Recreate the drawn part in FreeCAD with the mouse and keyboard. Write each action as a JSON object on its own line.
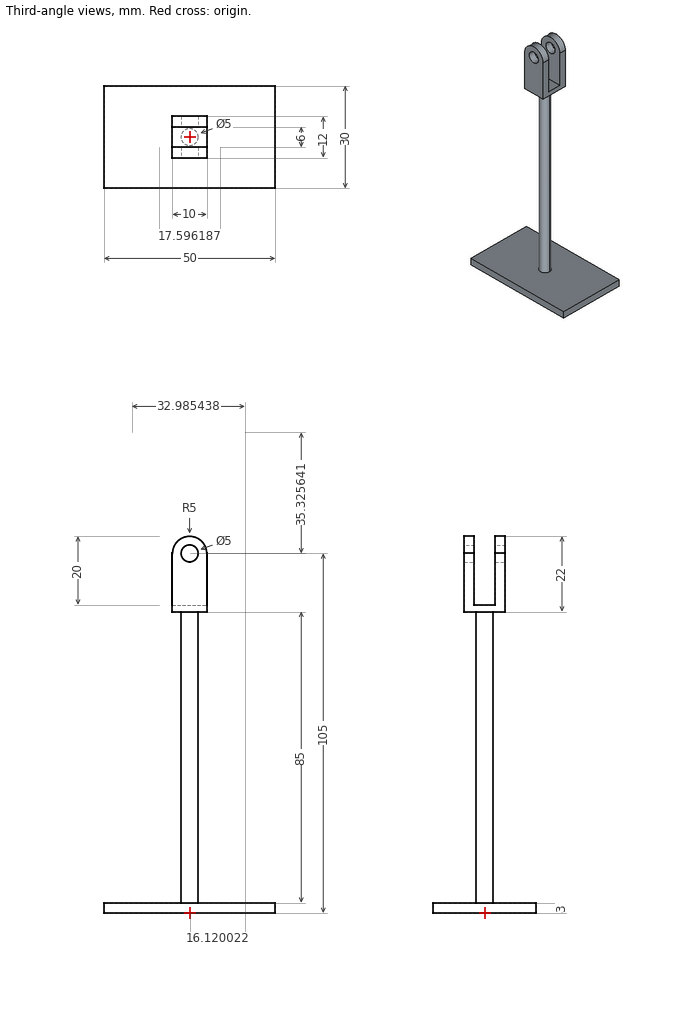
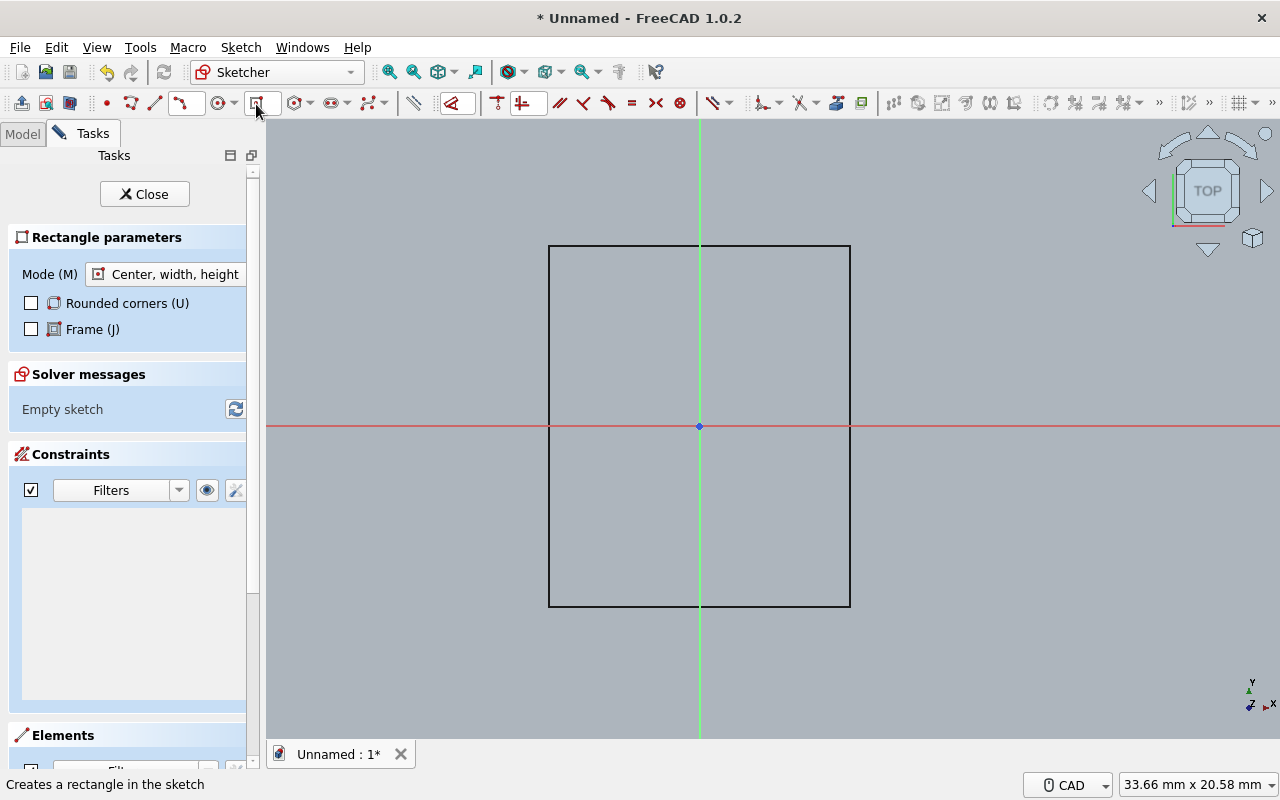
{"action": "left_click", "coordinate": [700, 426]}
{"action": "mouse_move", "coordinate": [965, 336]}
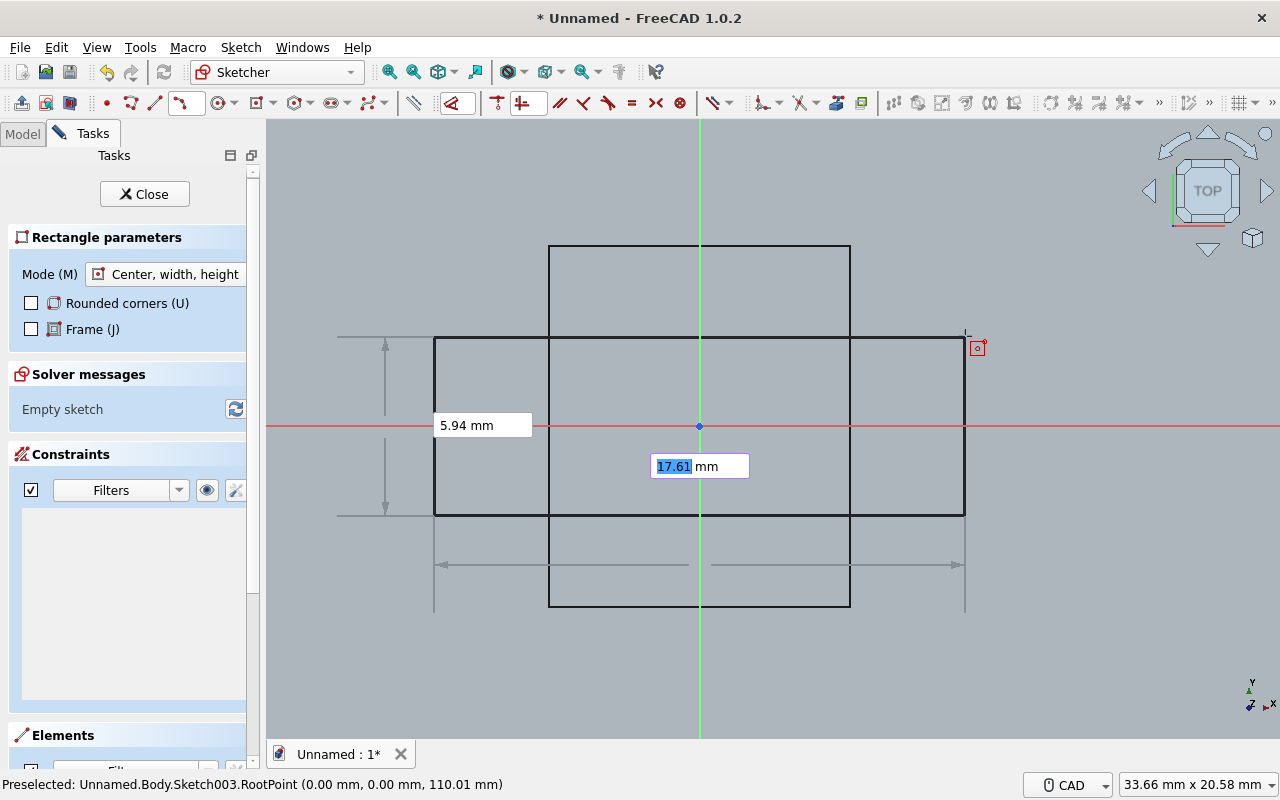
{"action": "type", "text": "17.596187"}
{"action": "key", "text": "Tab"}
{"action": "type", "text": "6"}
{"action": "key", "text": "Return"}
{"action": "key", "text": "Escape"}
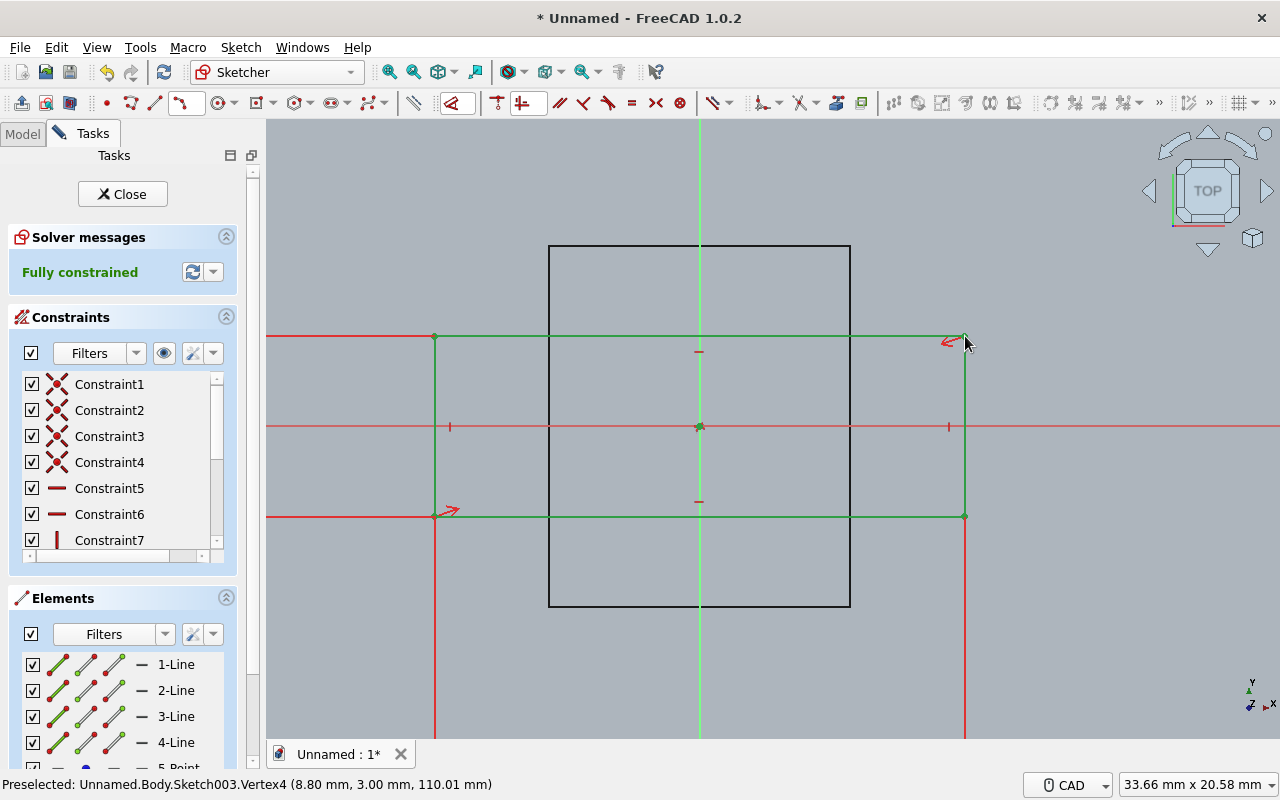
{"action": "left_click", "coordinate": [123, 194]}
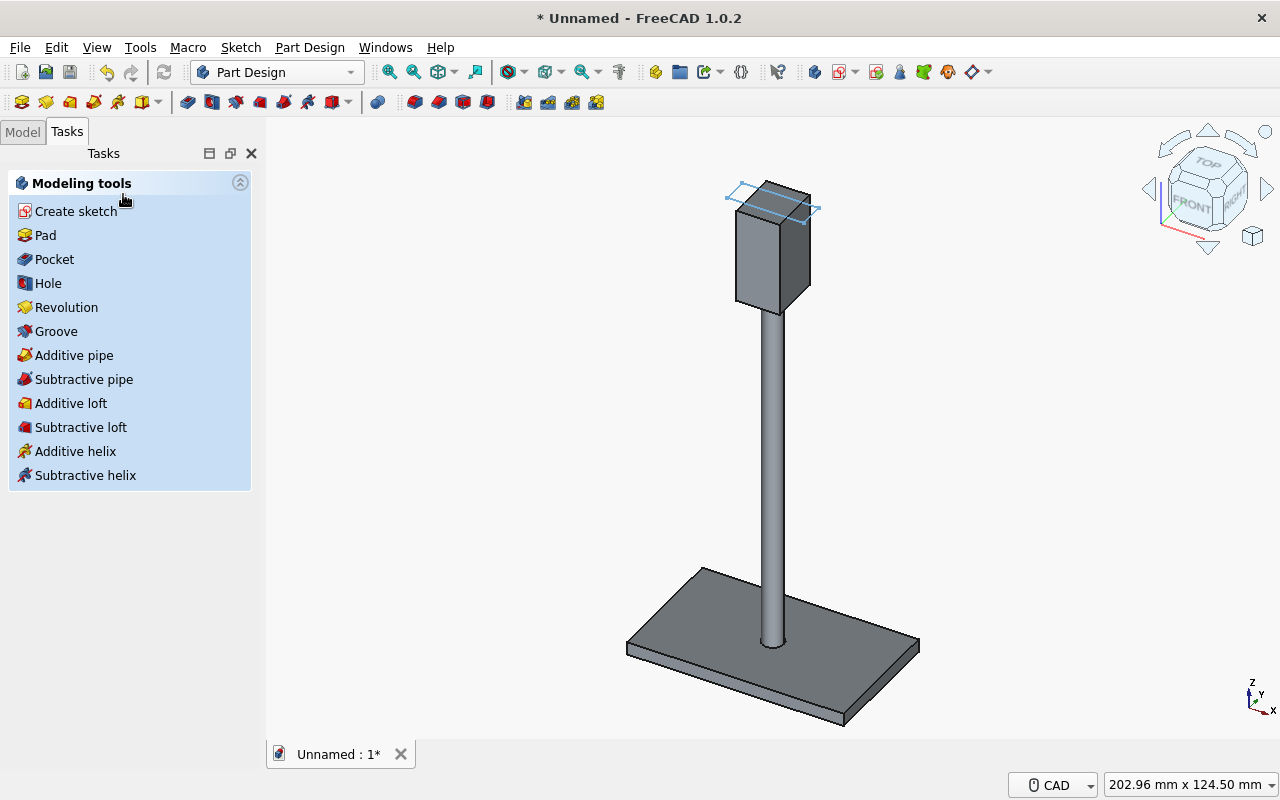
{"action": "left_click", "coordinate": [188, 102]}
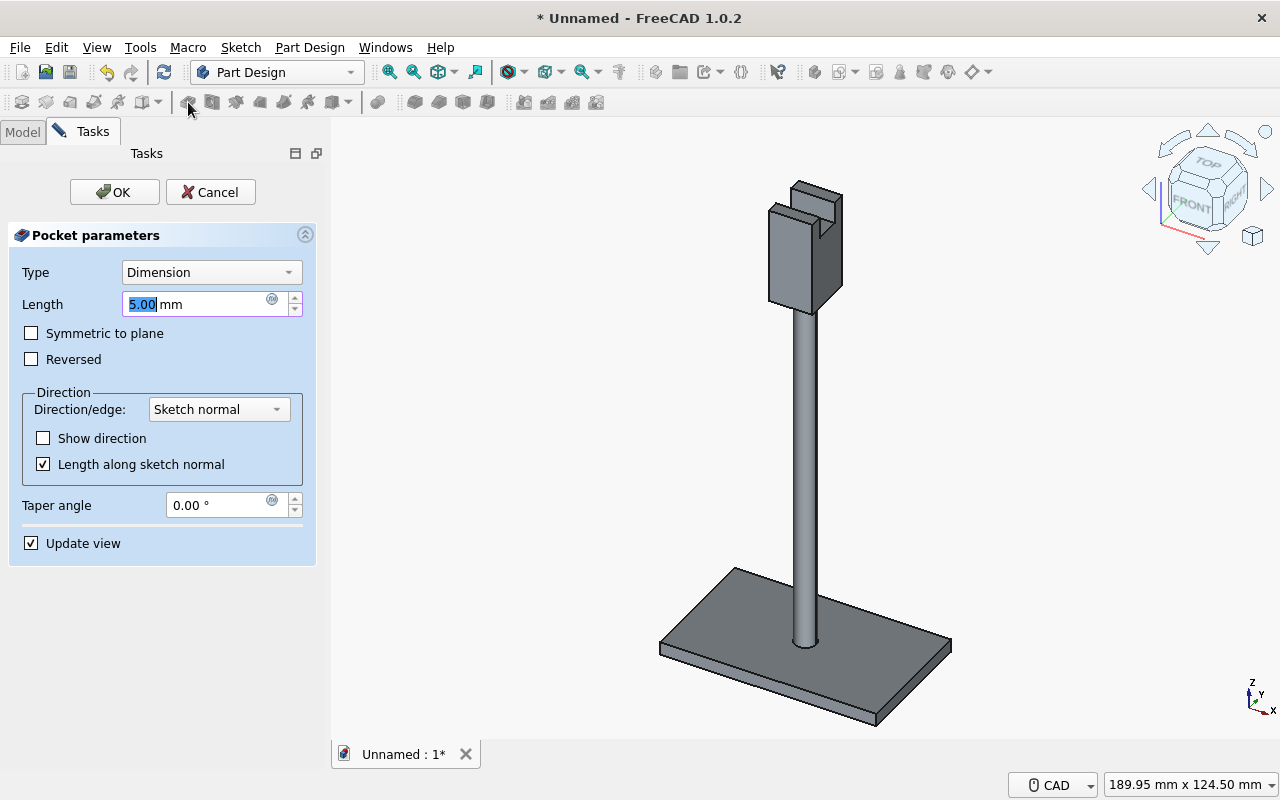
{"action": "type", "text": "20"}
{"action": "key", "text": "Tab"}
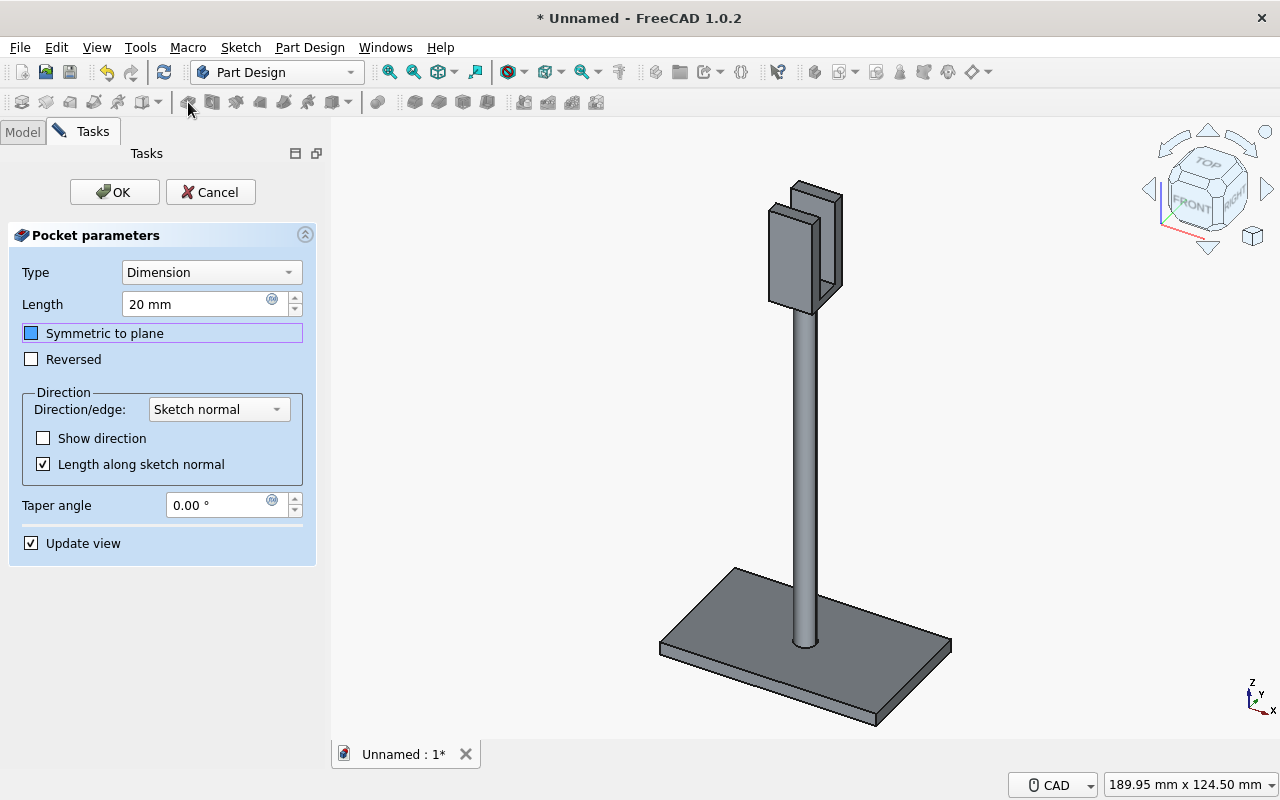
{"action": "left_click", "coordinate": [115, 192]}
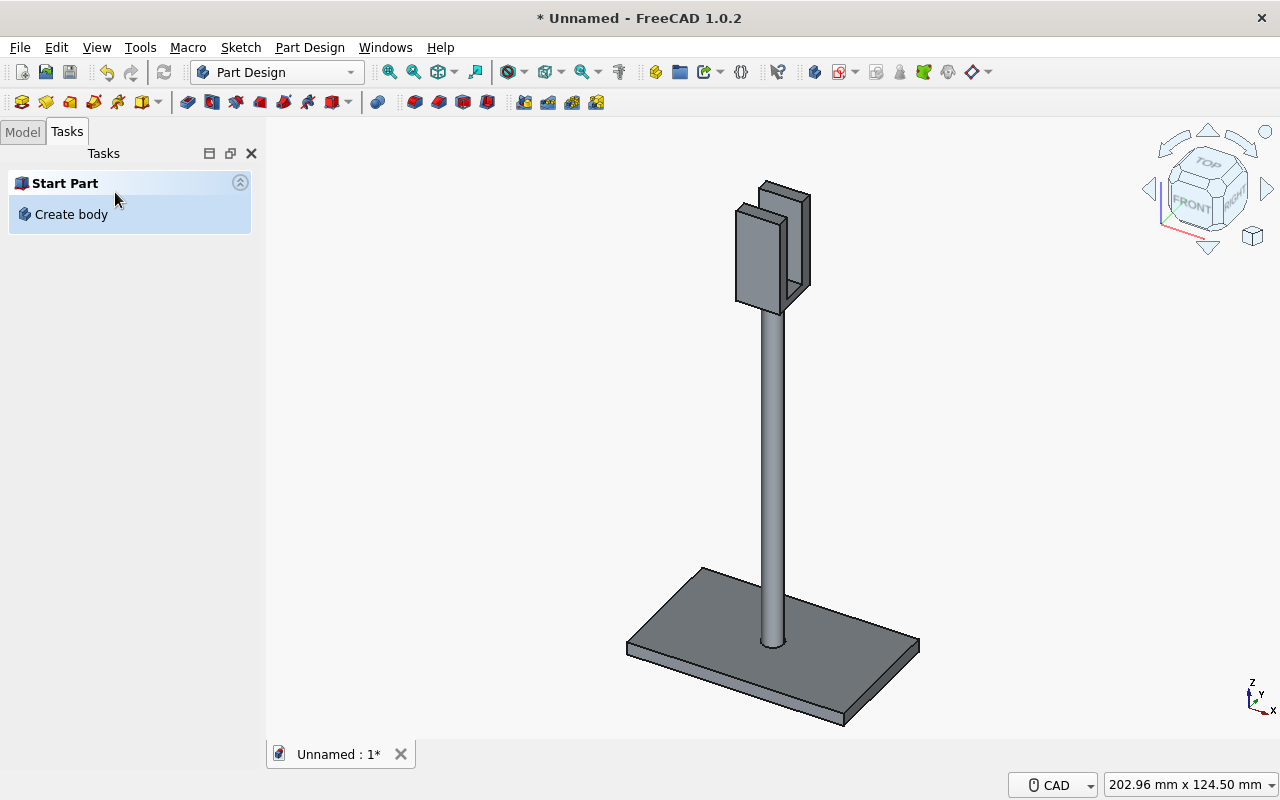
{"action": "left_click", "coordinate": [758, 249]}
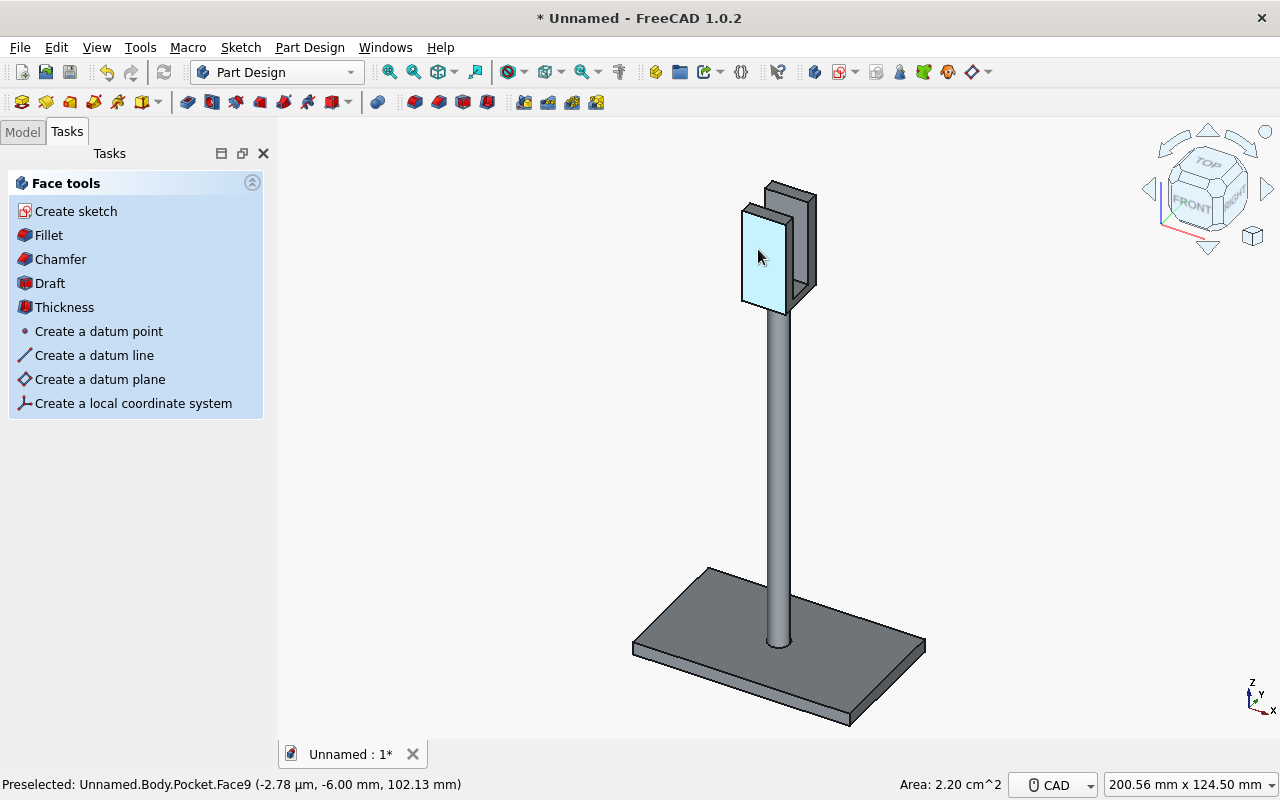
{"action": "left_click", "coordinate": [840, 72]}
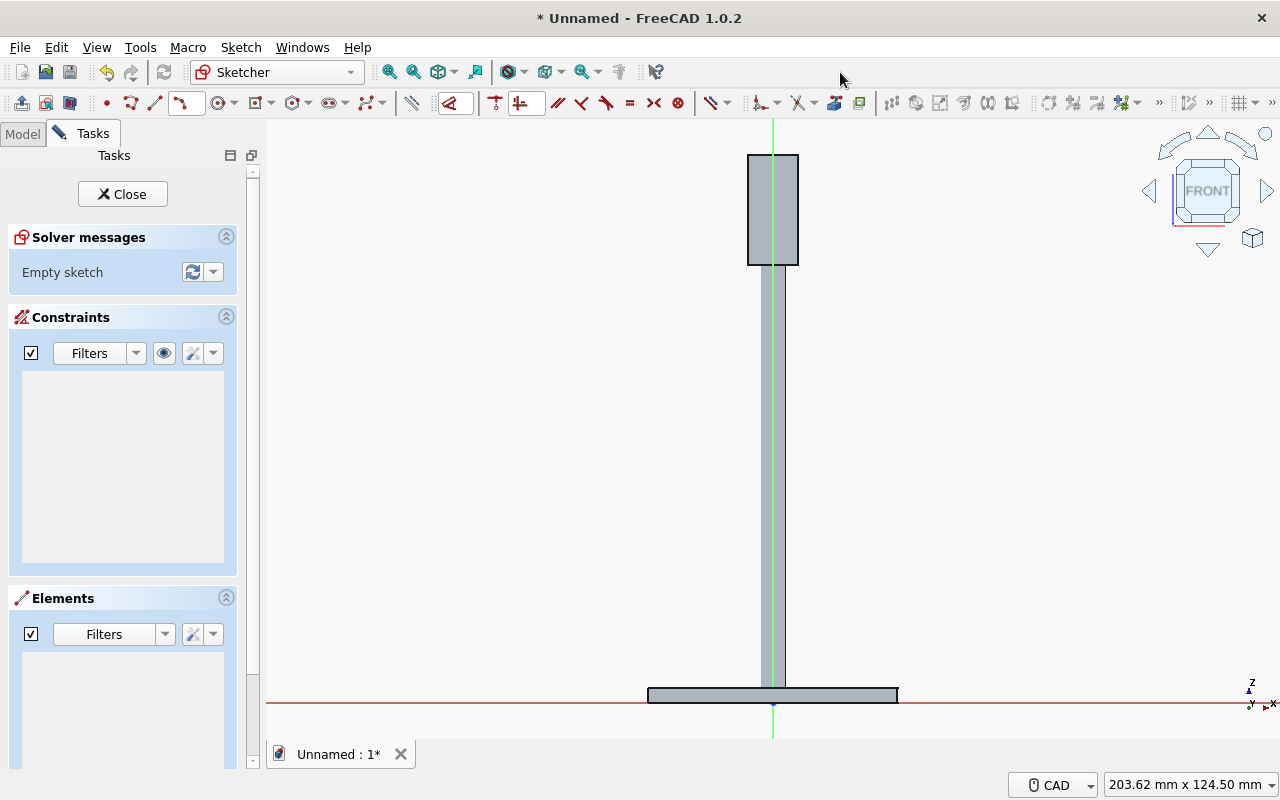
{"action": "left_click", "coordinate": [70, 104]}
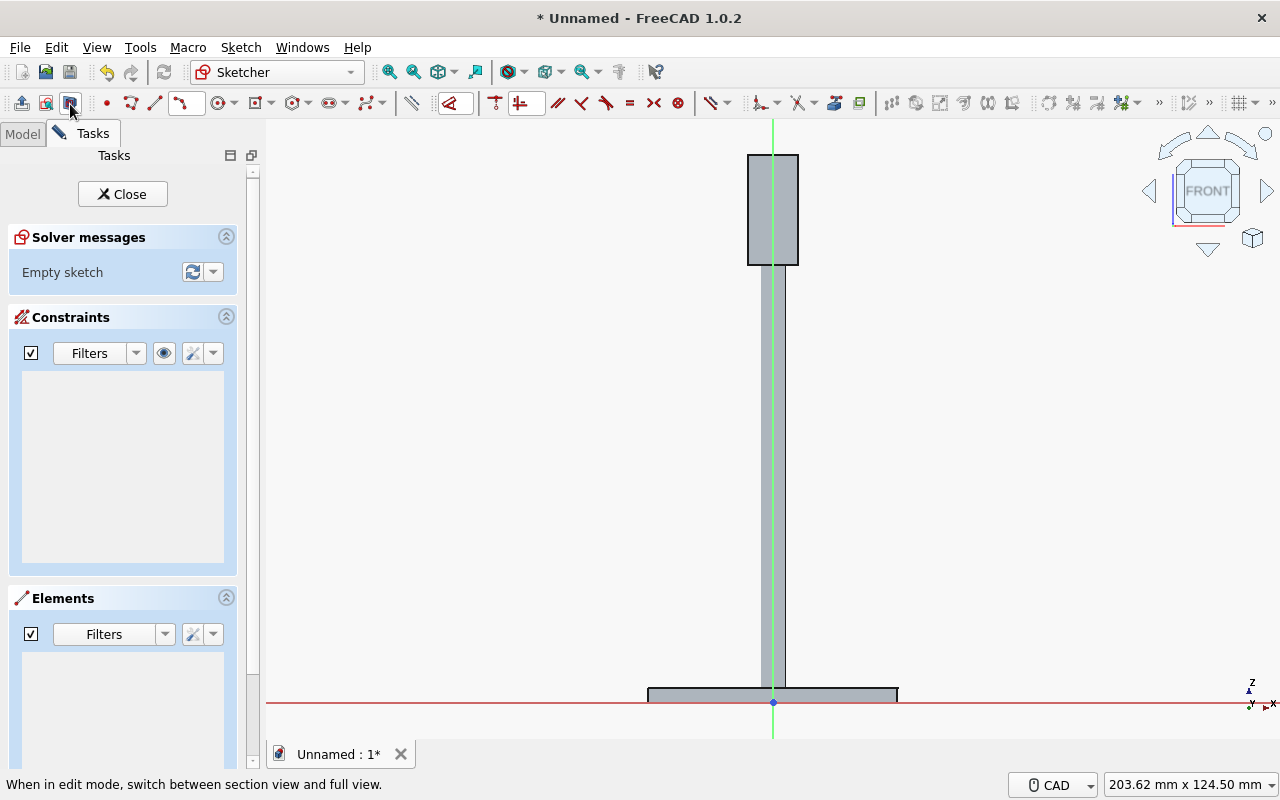
{"action": "scroll", "coordinate": [704, 429], "scroll_direction": "down", "scroll_amount": 5}